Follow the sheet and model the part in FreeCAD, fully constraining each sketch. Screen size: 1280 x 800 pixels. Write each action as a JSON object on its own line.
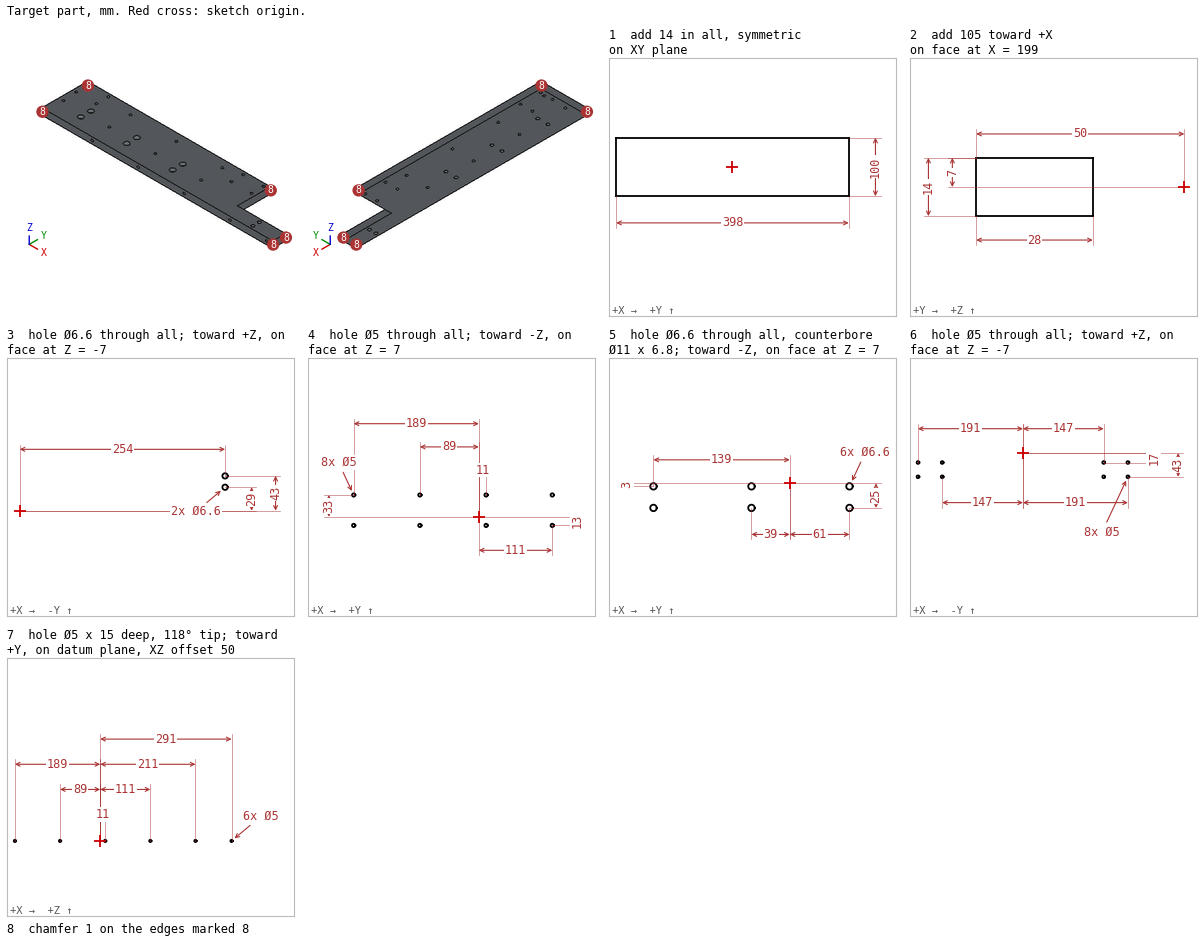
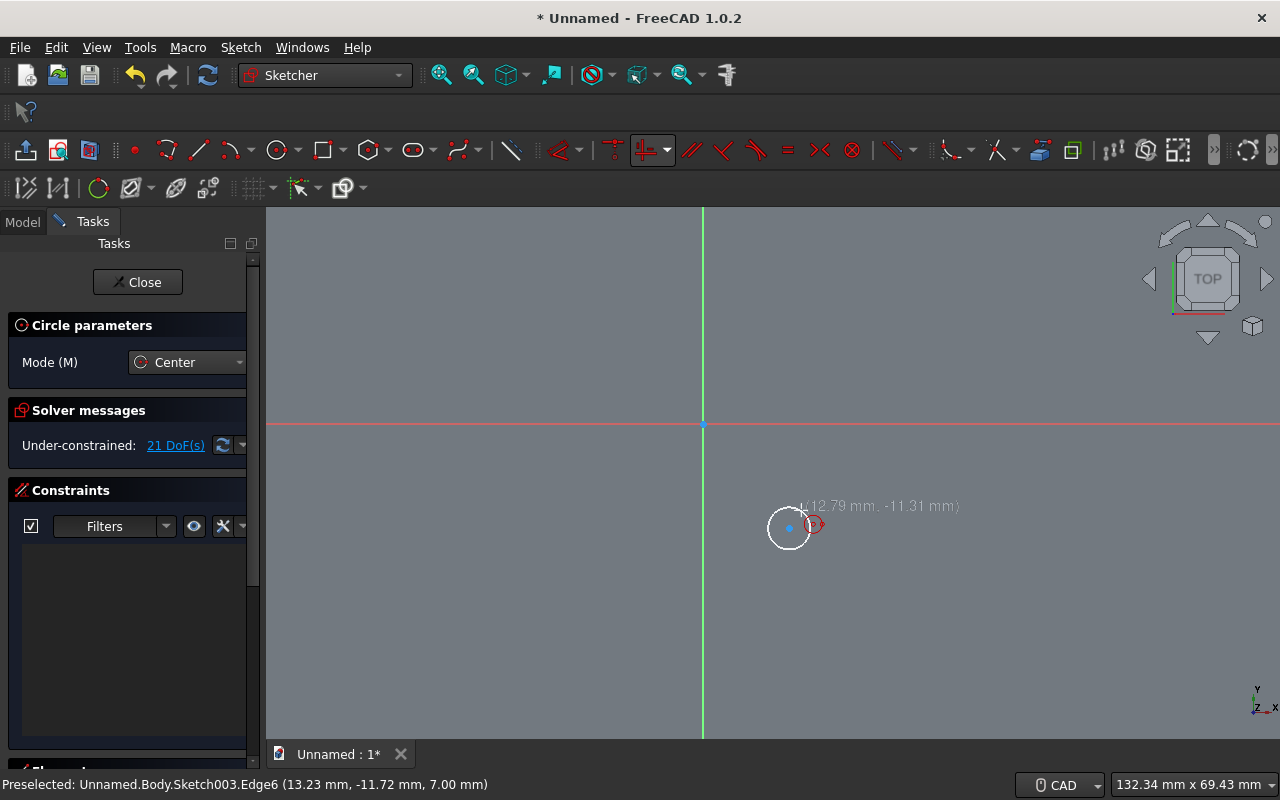
{"action": "scroll", "coordinate": [803, 514], "scroll_direction": "down", "scroll_amount": 7}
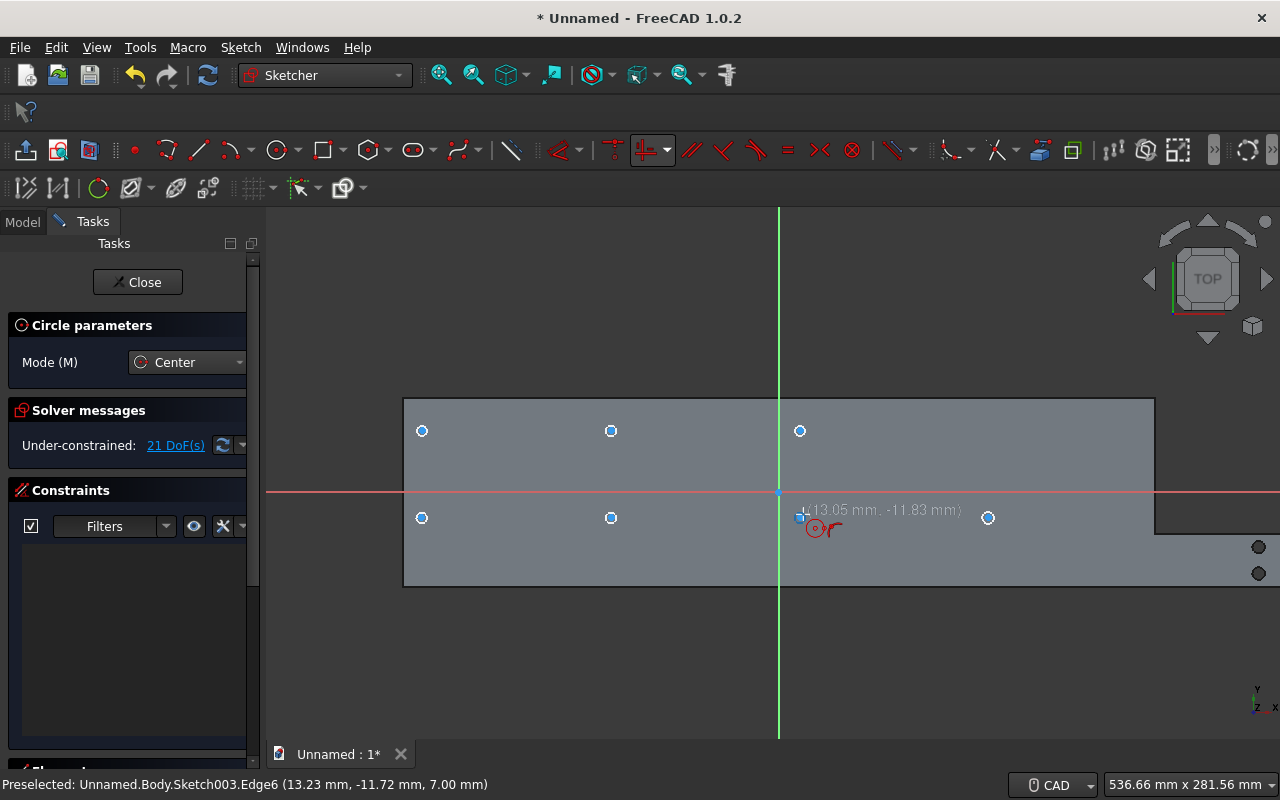
{"action": "scroll", "coordinate": [988, 430], "scroll_direction": "up", "scroll_amount": 8}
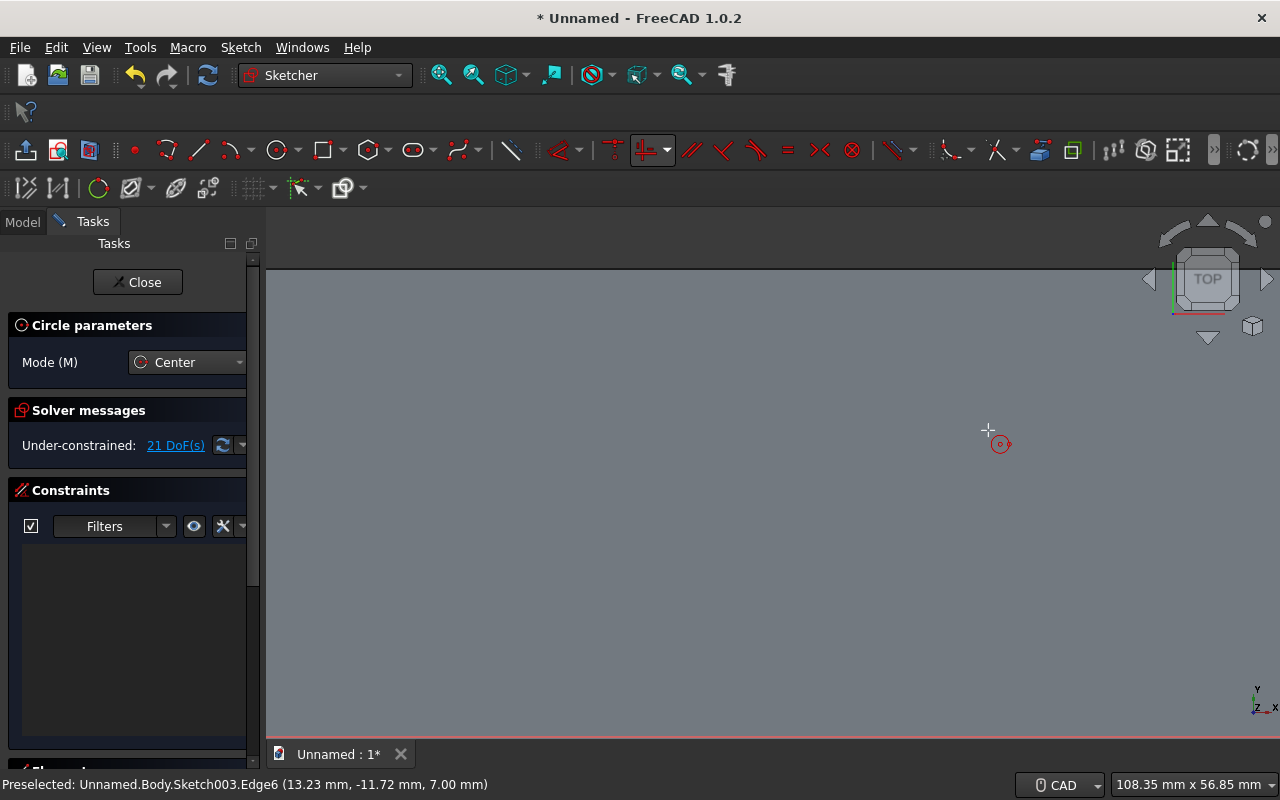
{"action": "scroll", "coordinate": [988, 430], "scroll_direction": "down", "scroll_amount": 8}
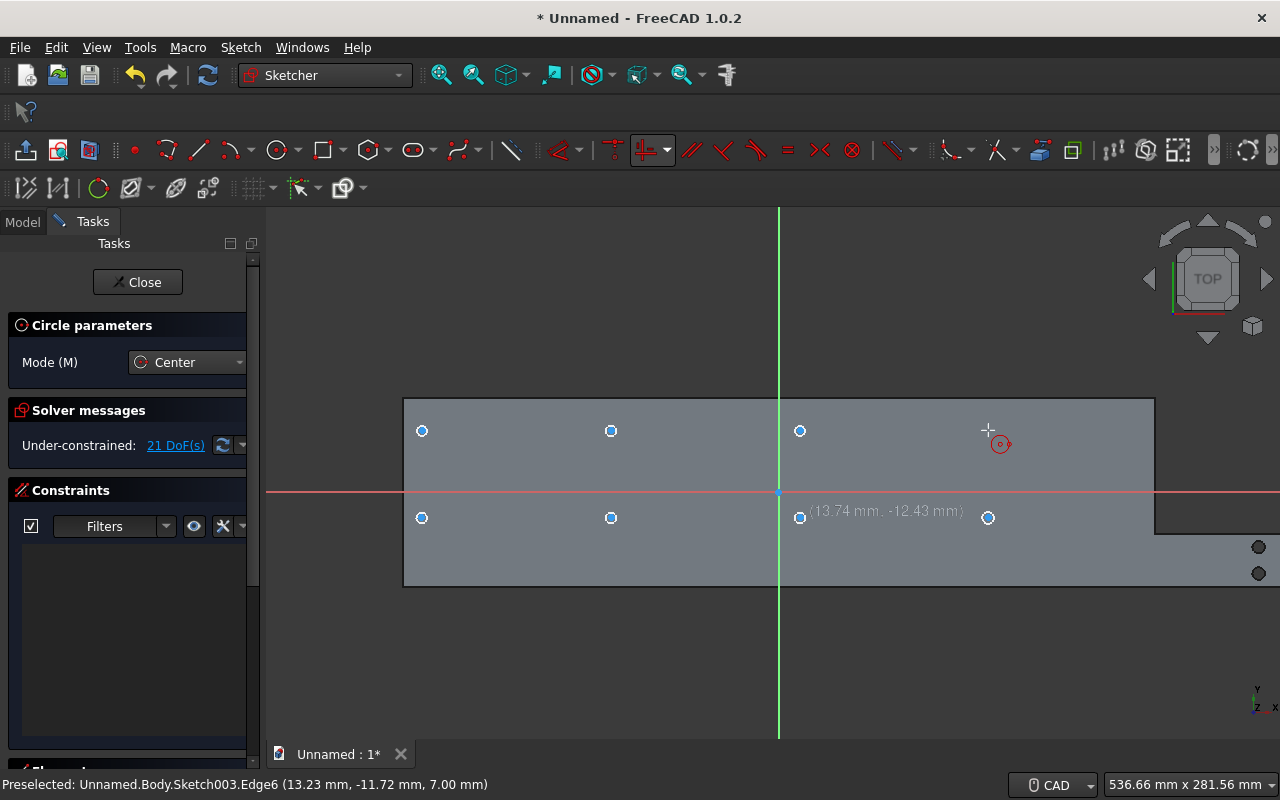
{"action": "left_click", "coordinate": [988, 430]}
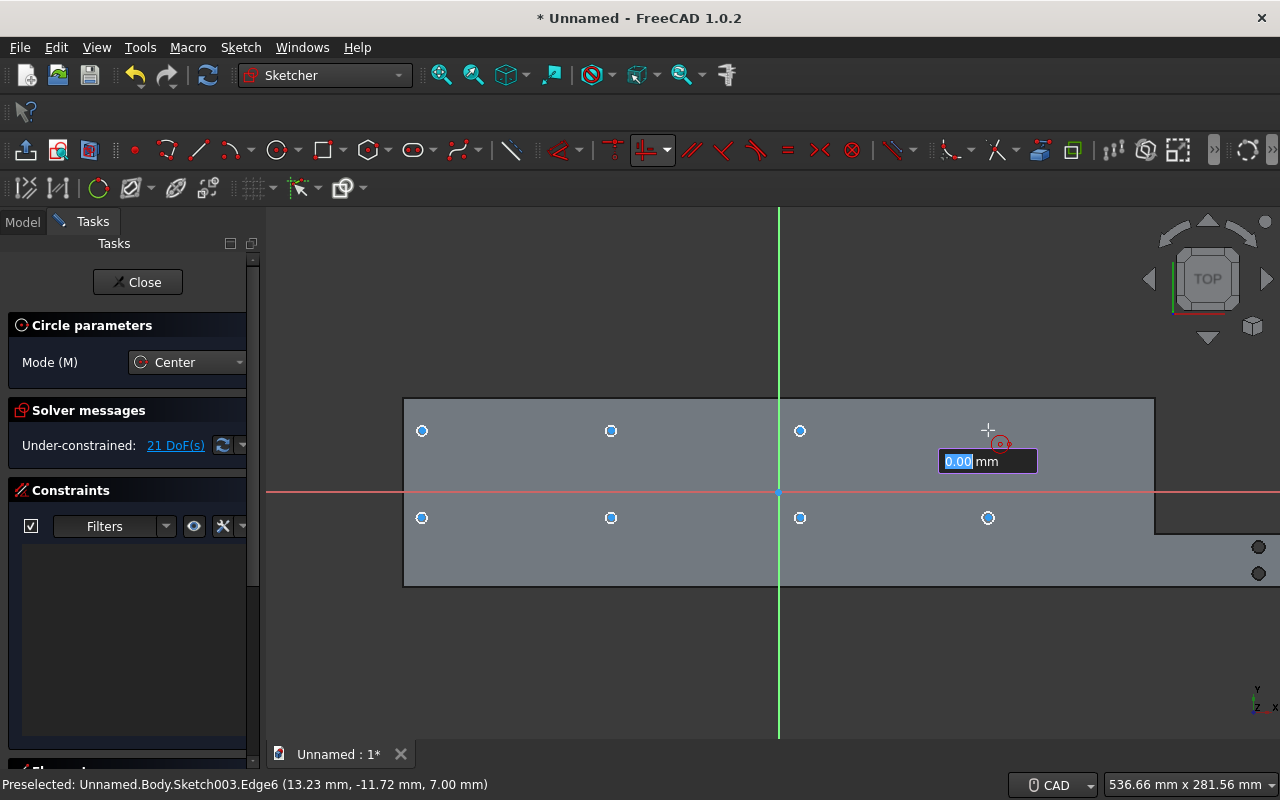
{"action": "scroll", "coordinate": [992, 427], "scroll_direction": "up", "scroll_amount": 7}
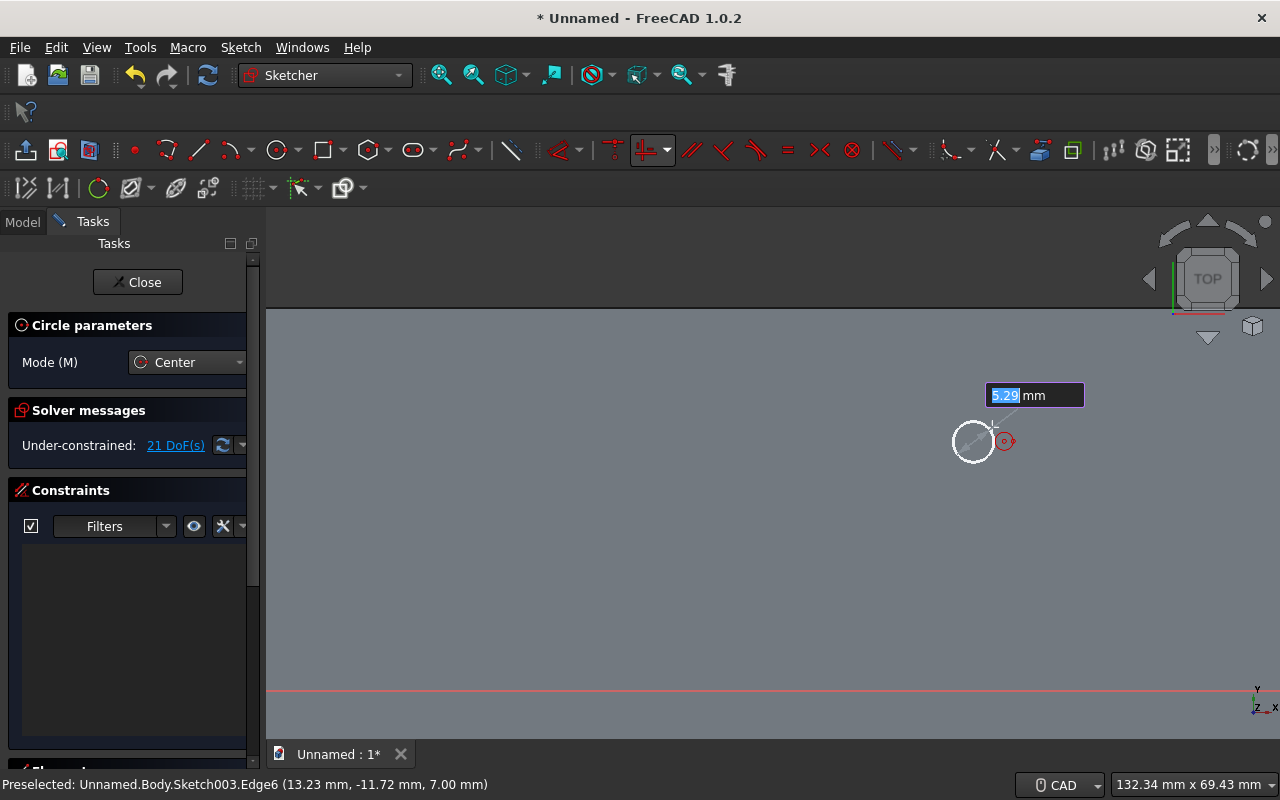
{"action": "left_click", "coordinate": [989, 424]}
{"action": "key", "text": "Escape"}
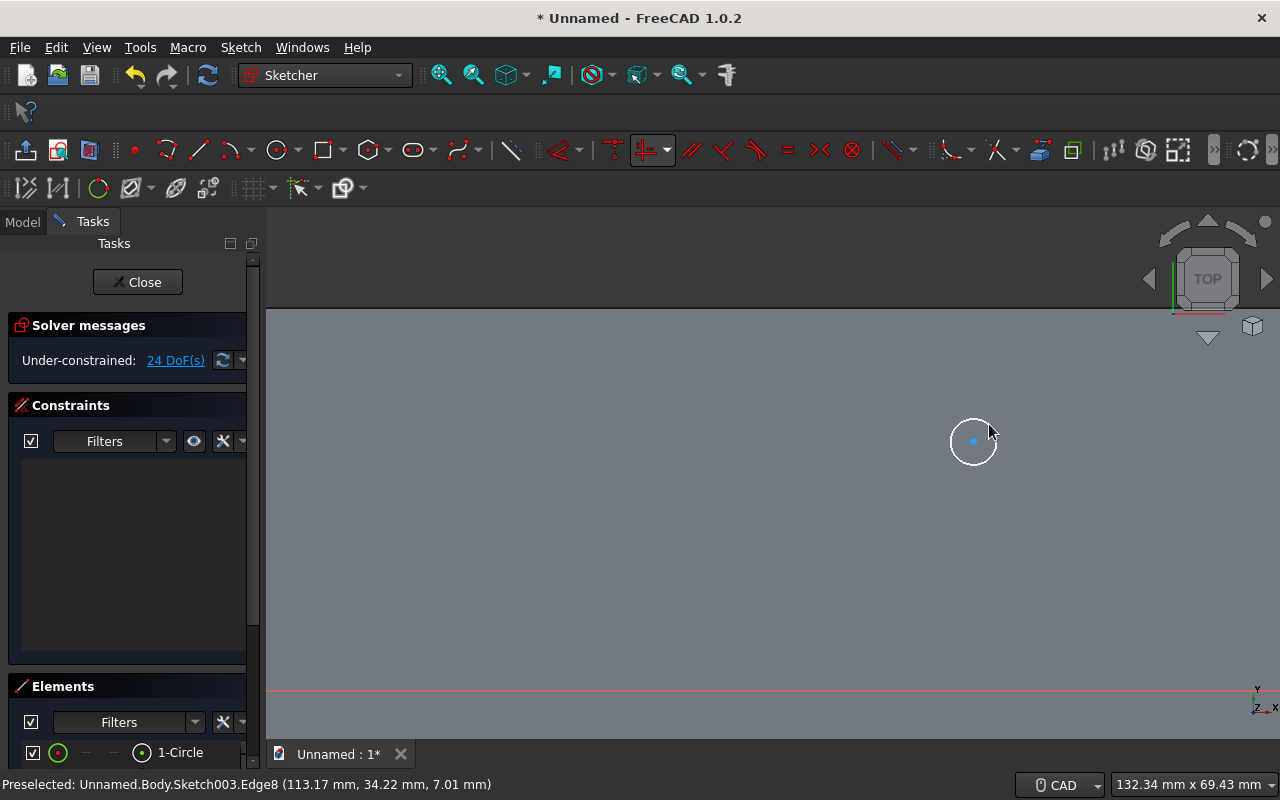
{"action": "scroll", "coordinate": [992, 427], "scroll_direction": "down", "scroll_amount": 7}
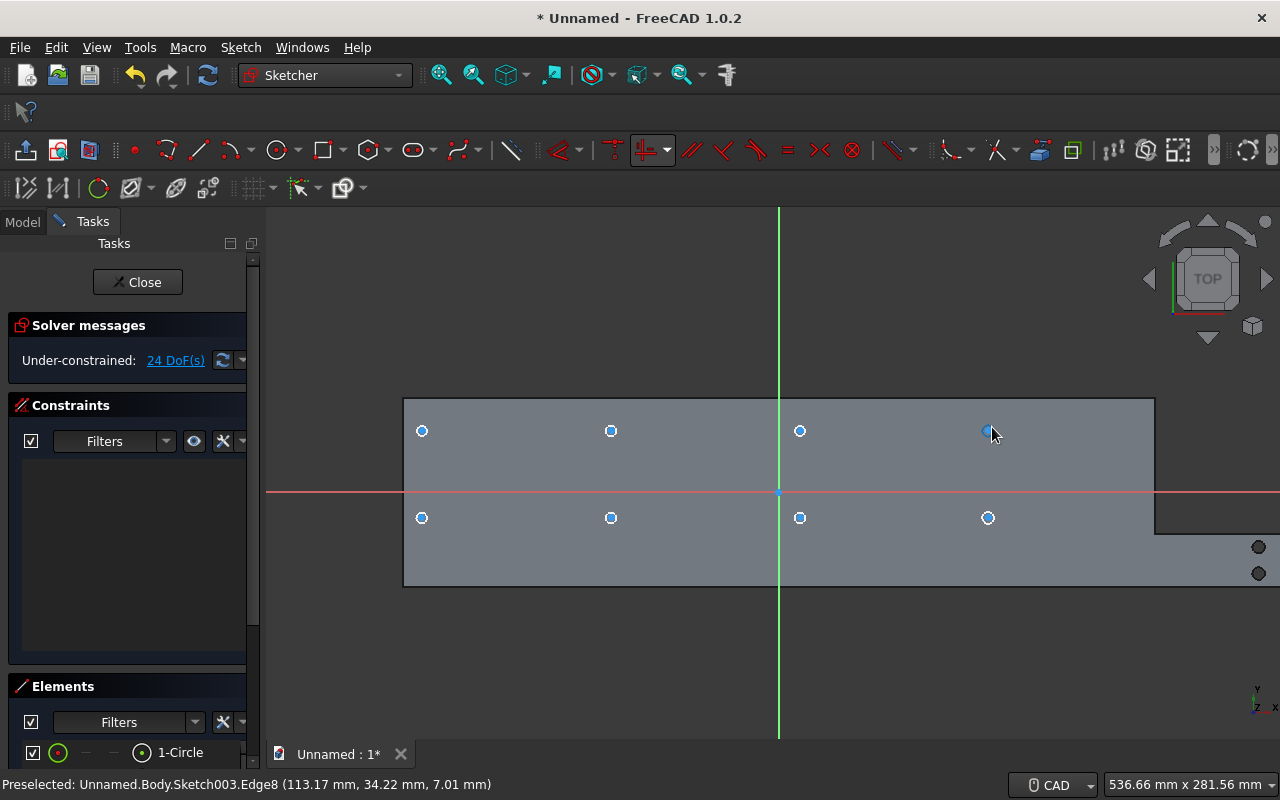
{"action": "scroll", "coordinate": [992, 514], "scroll_direction": "up", "scroll_amount": 5}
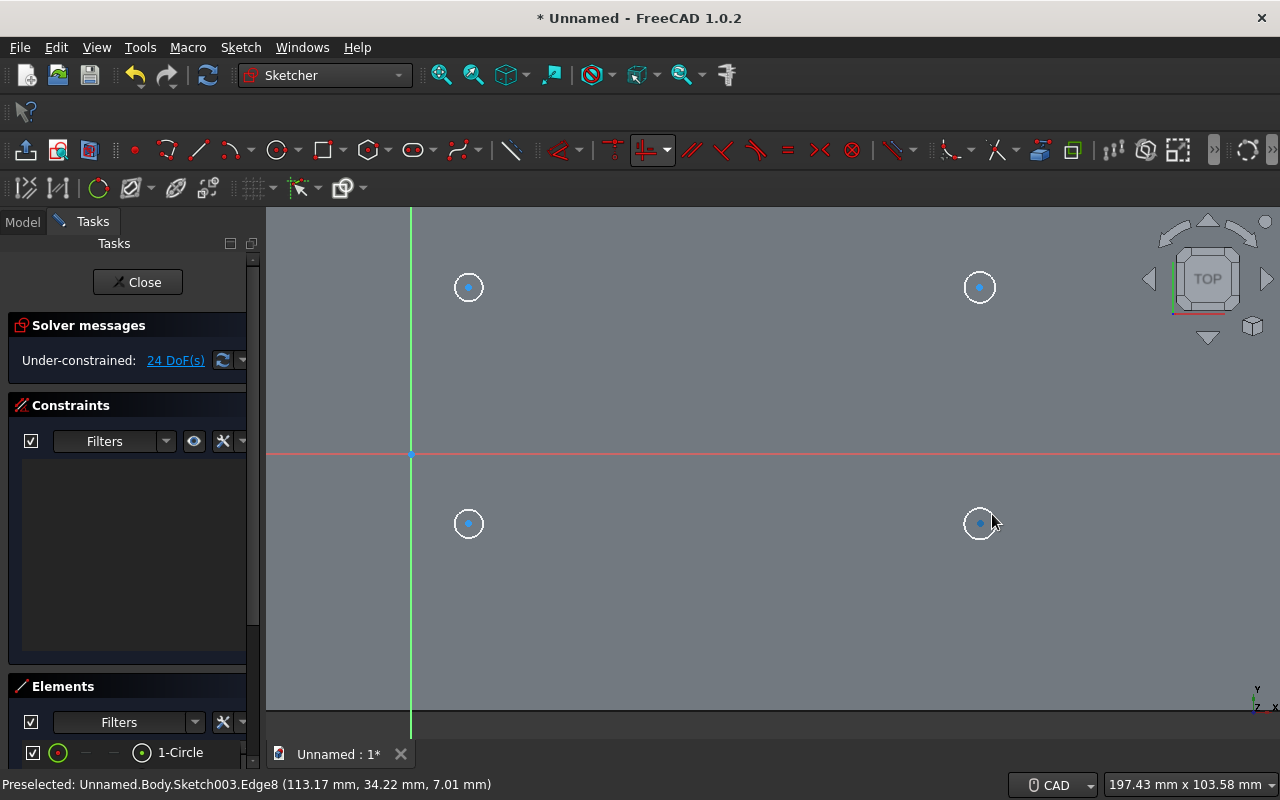
{"action": "left_click", "coordinate": [991, 513]}